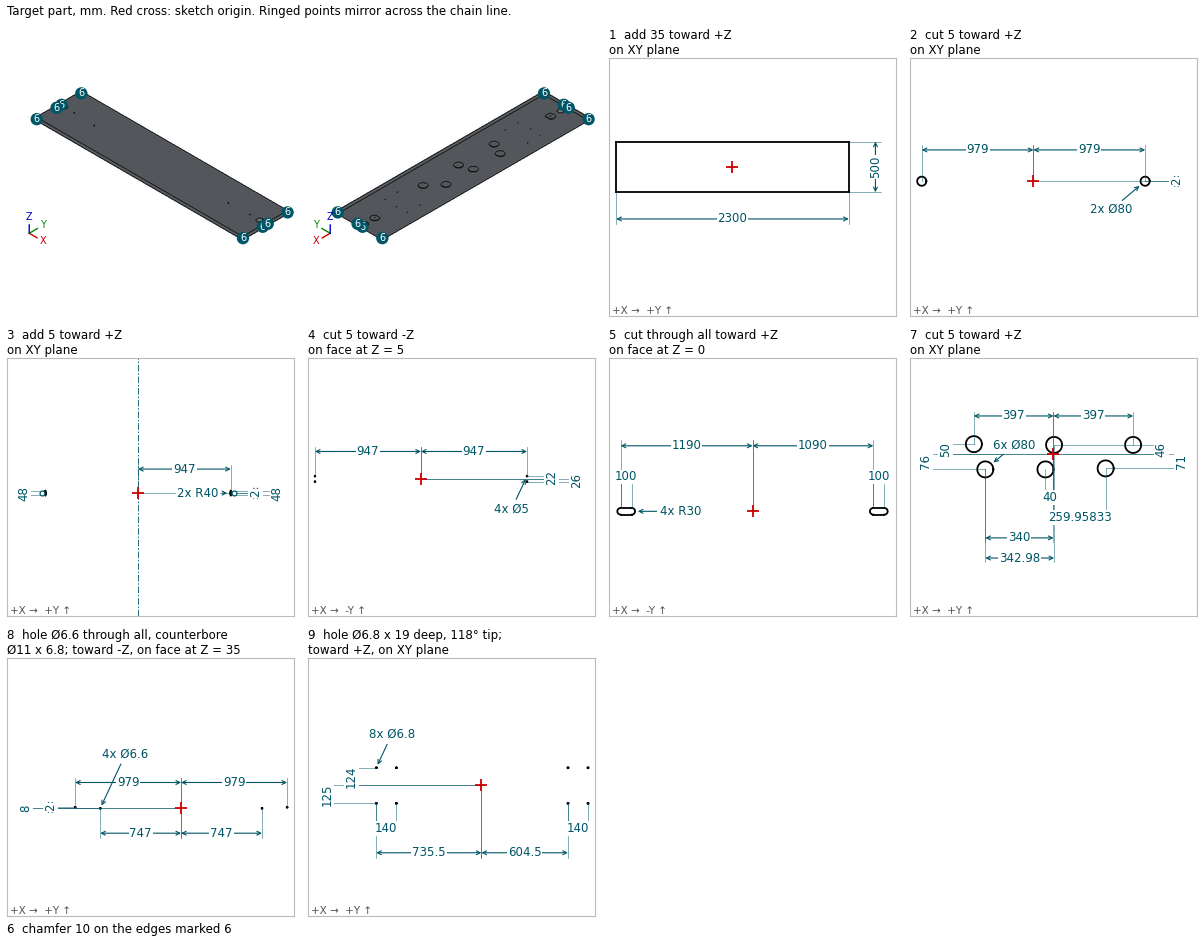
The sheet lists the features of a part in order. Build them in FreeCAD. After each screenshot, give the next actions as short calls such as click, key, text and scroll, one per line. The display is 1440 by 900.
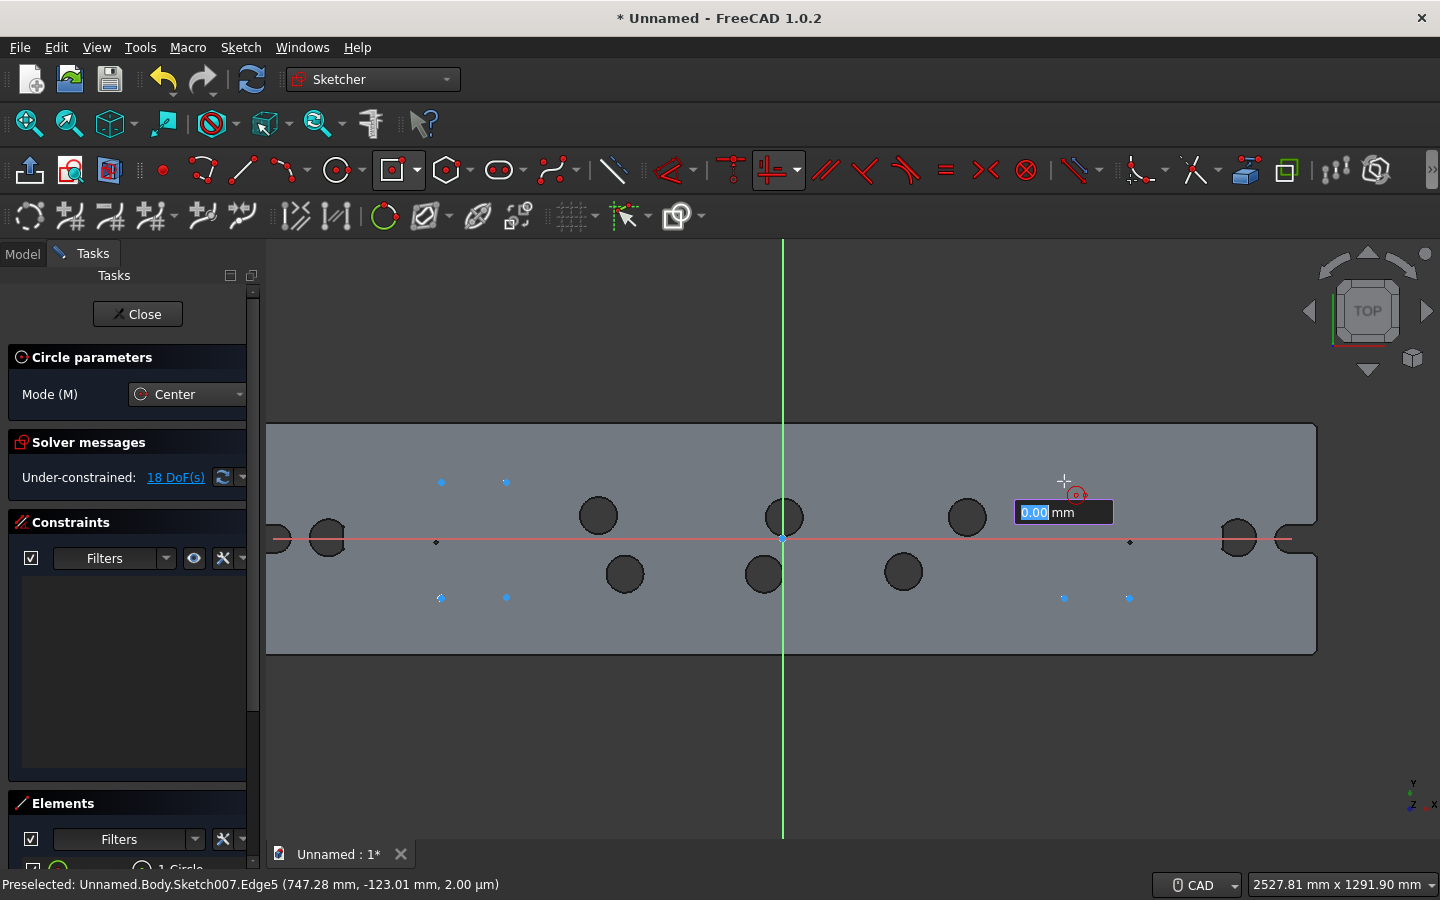
scroll(1065, 480, up, 12)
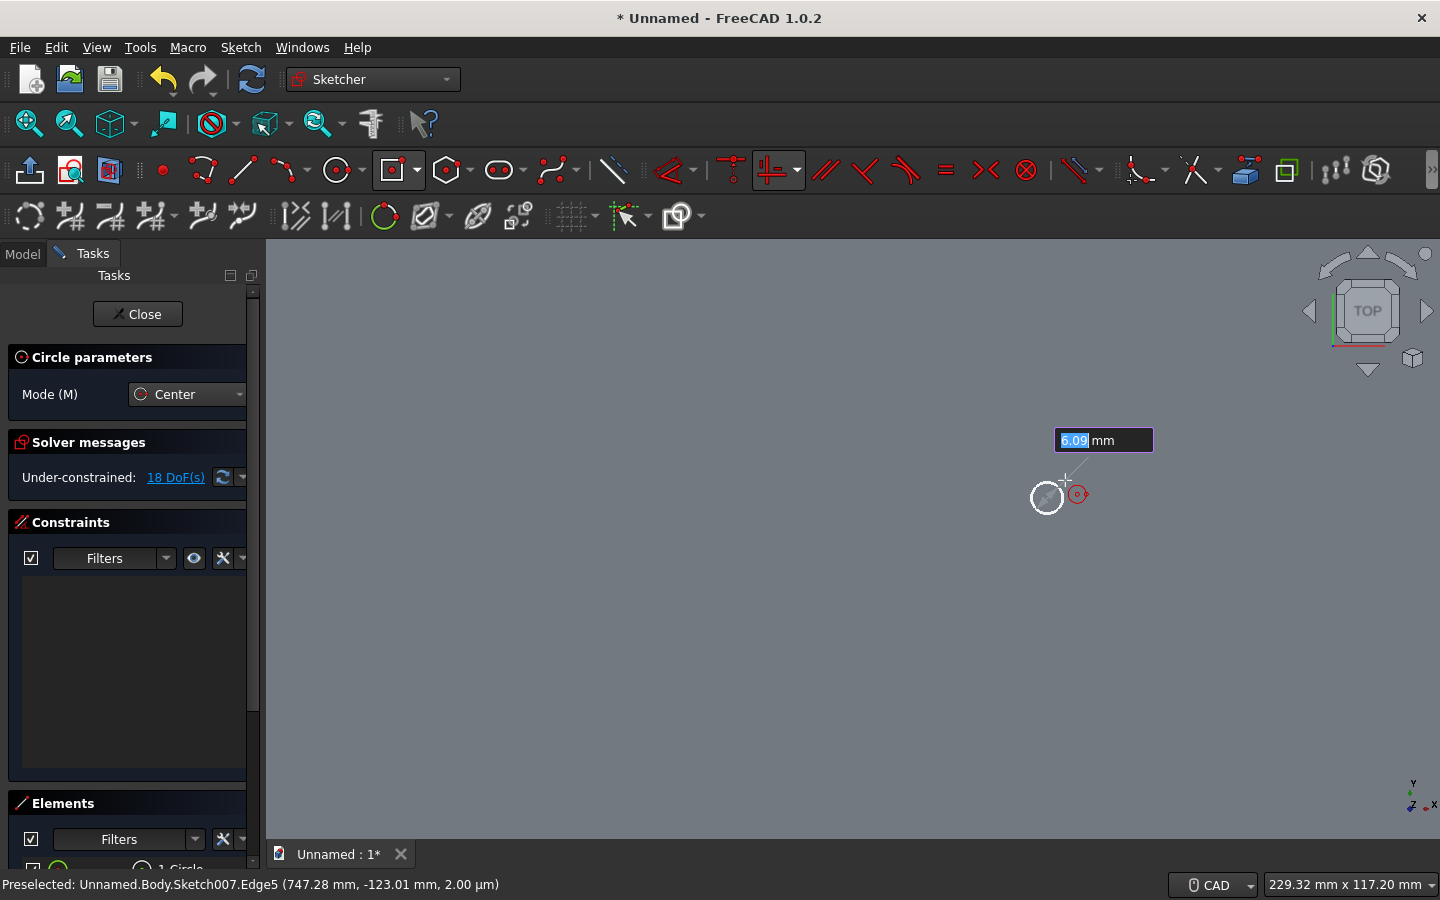
click(1056, 477)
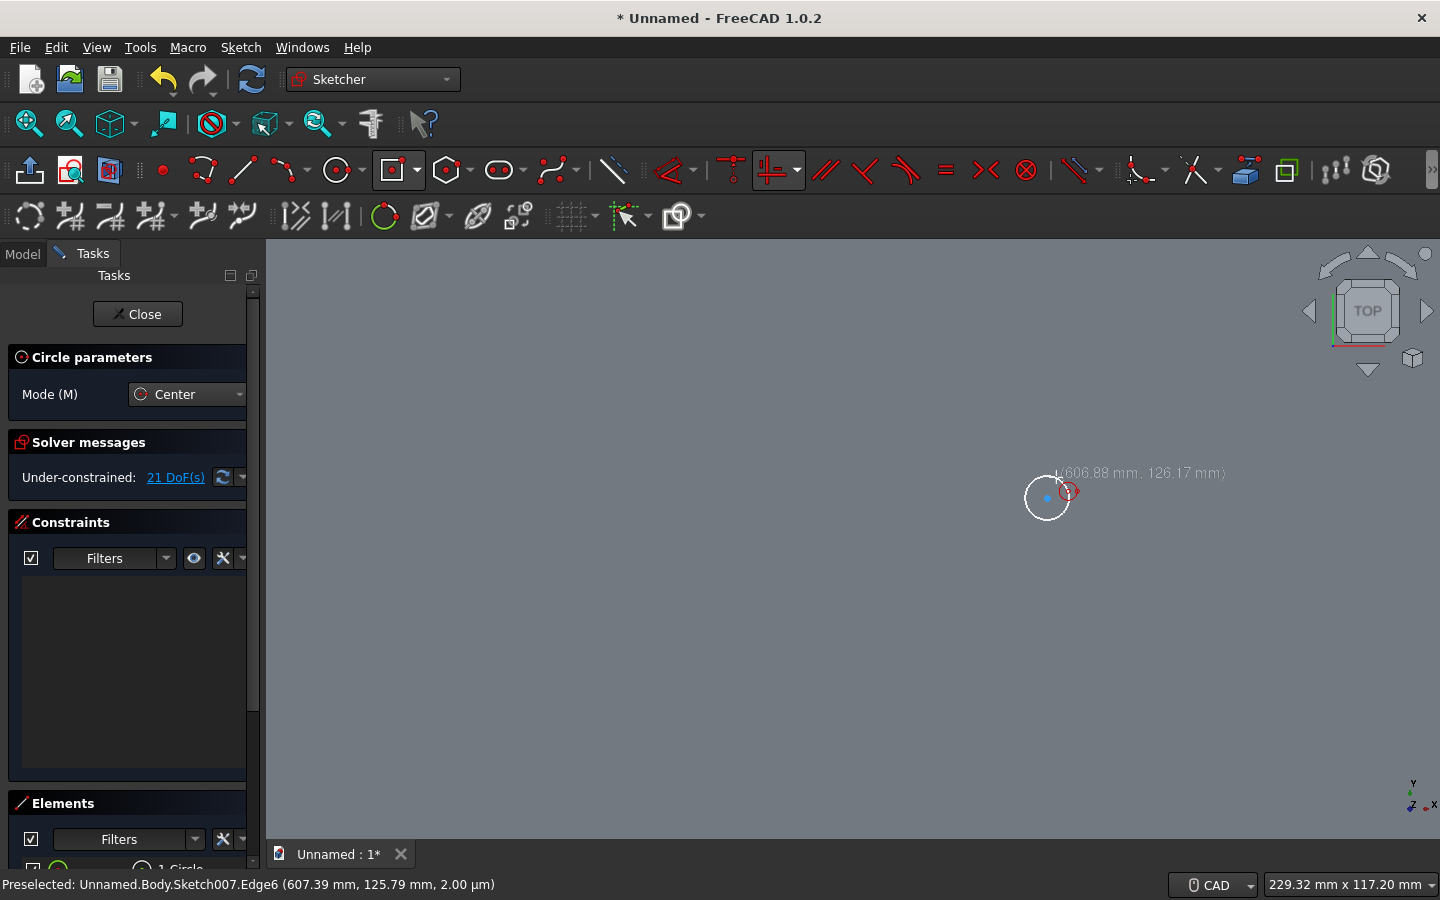
scroll(1065, 480, down, 12)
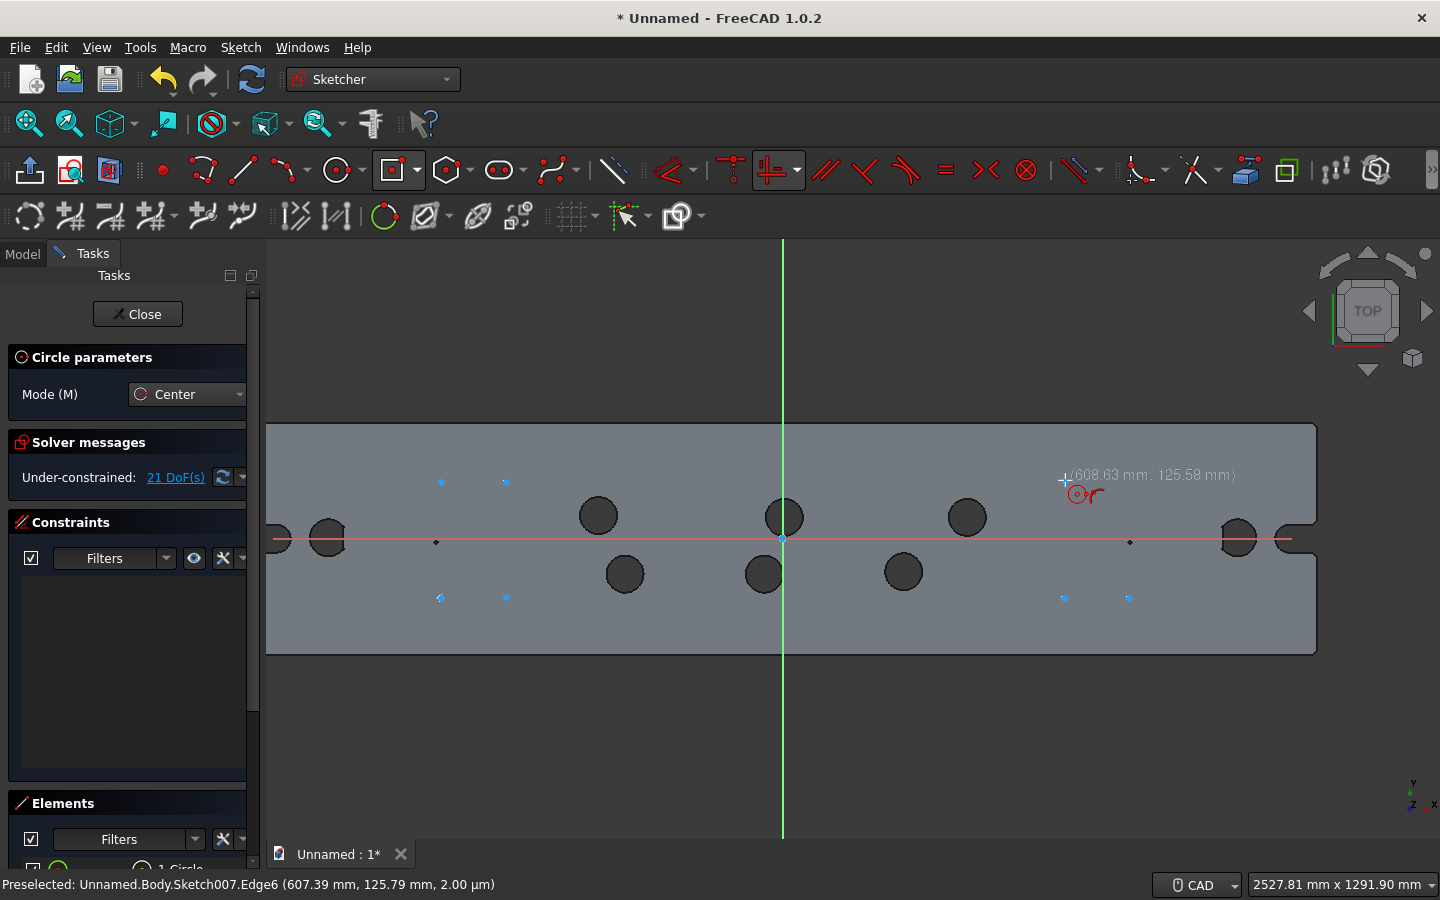
scroll(1129, 481, up, 14)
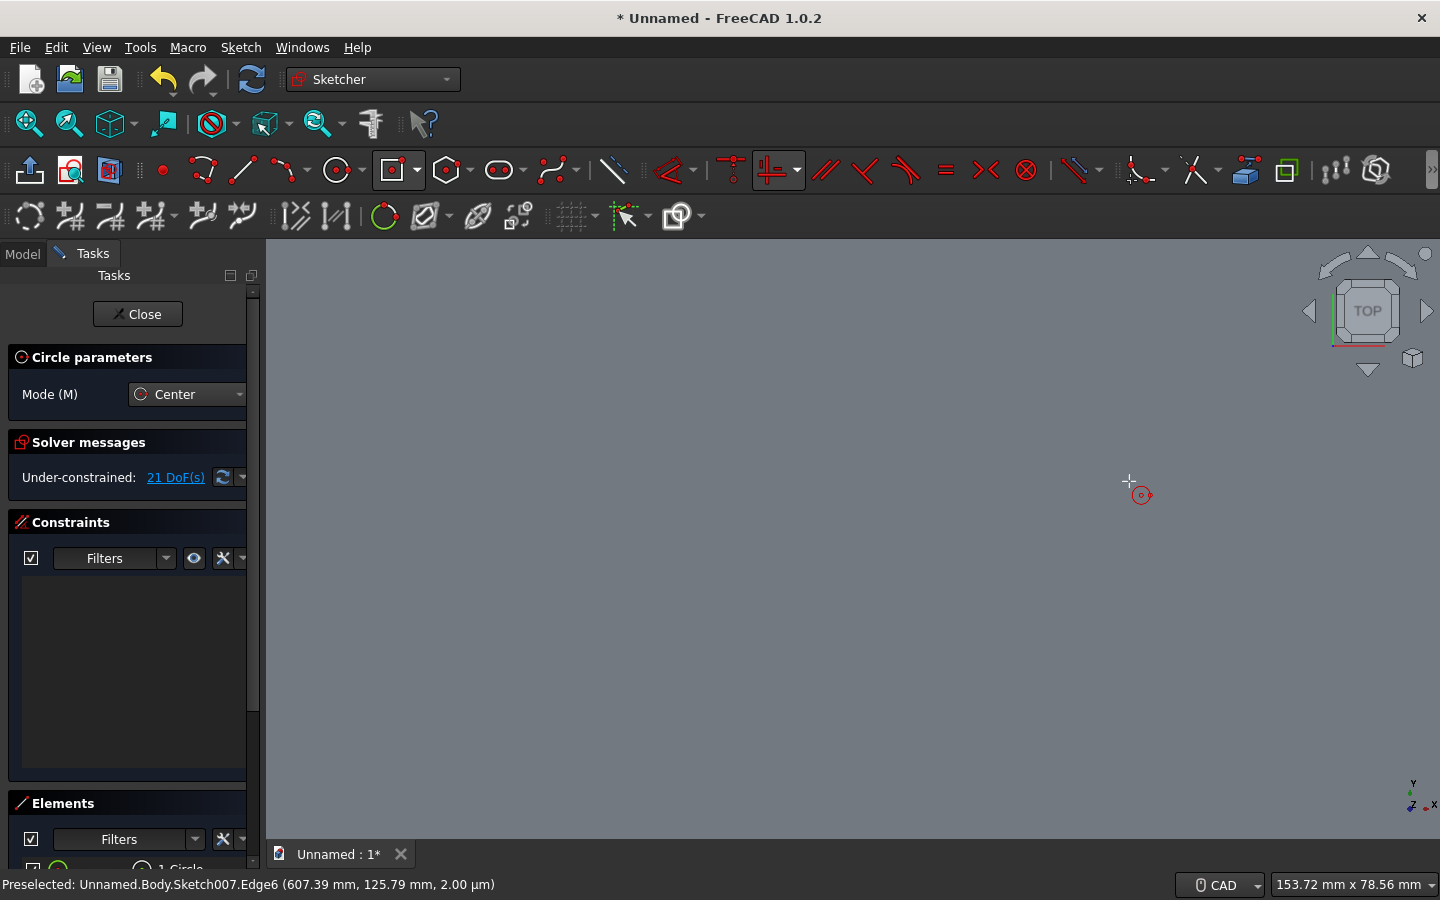
scroll(1129, 481, down, 14)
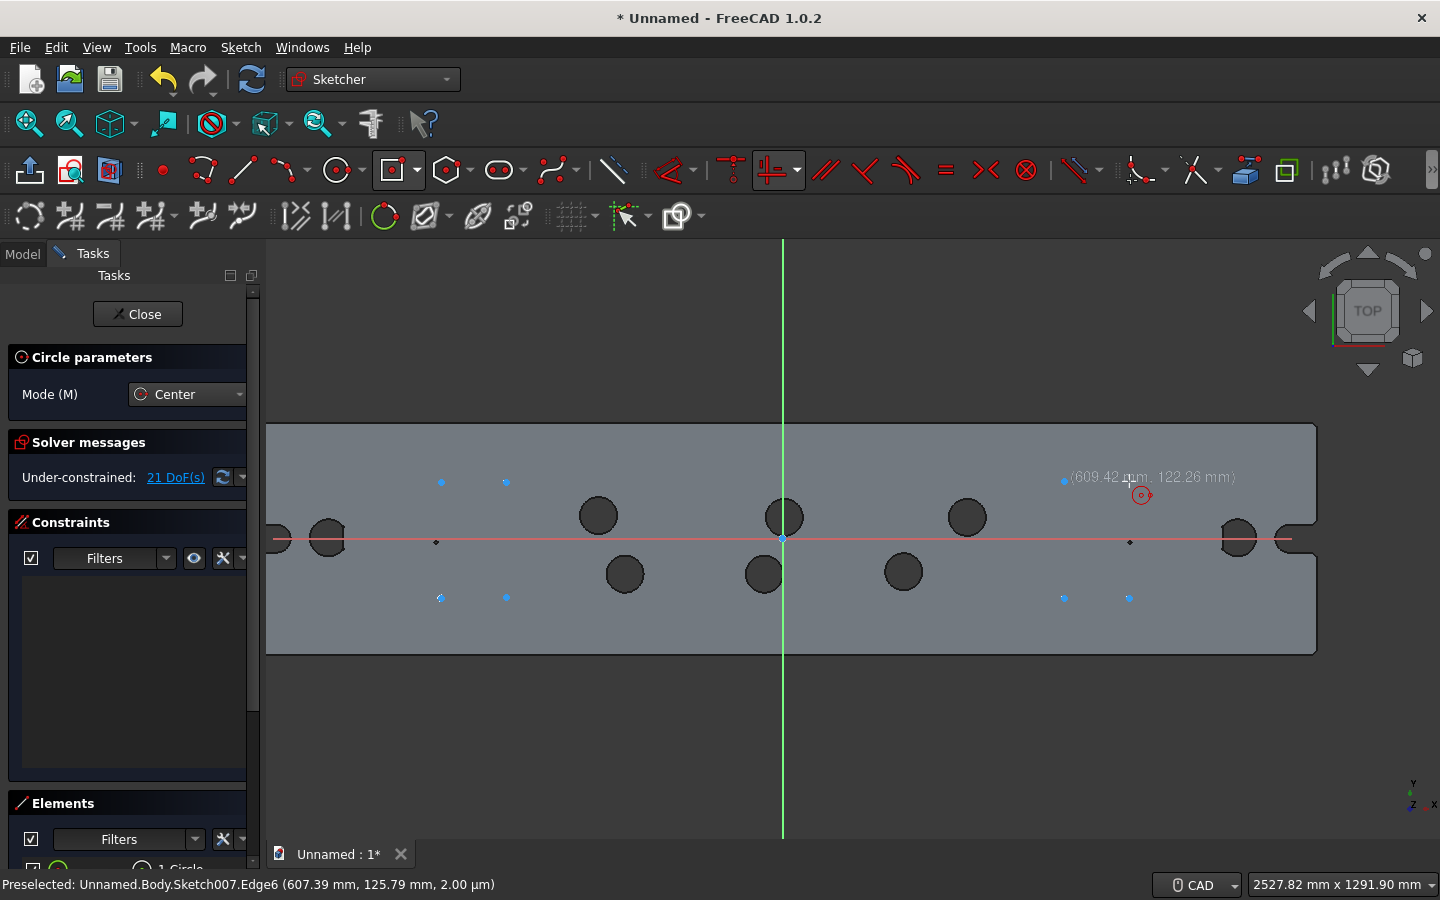
click(1129, 481)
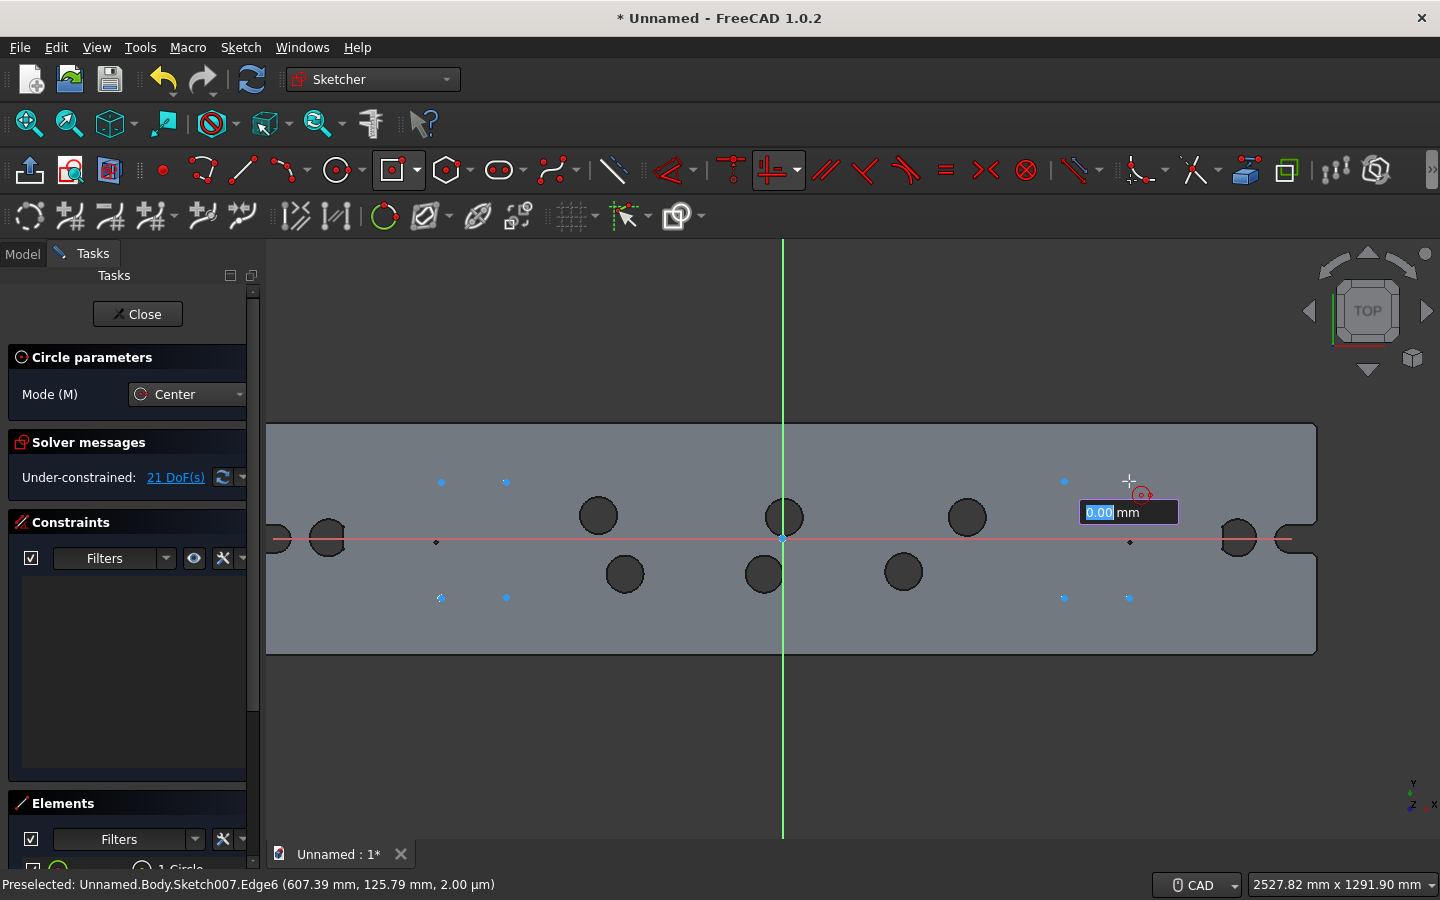
scroll(1130, 480, up, 12)